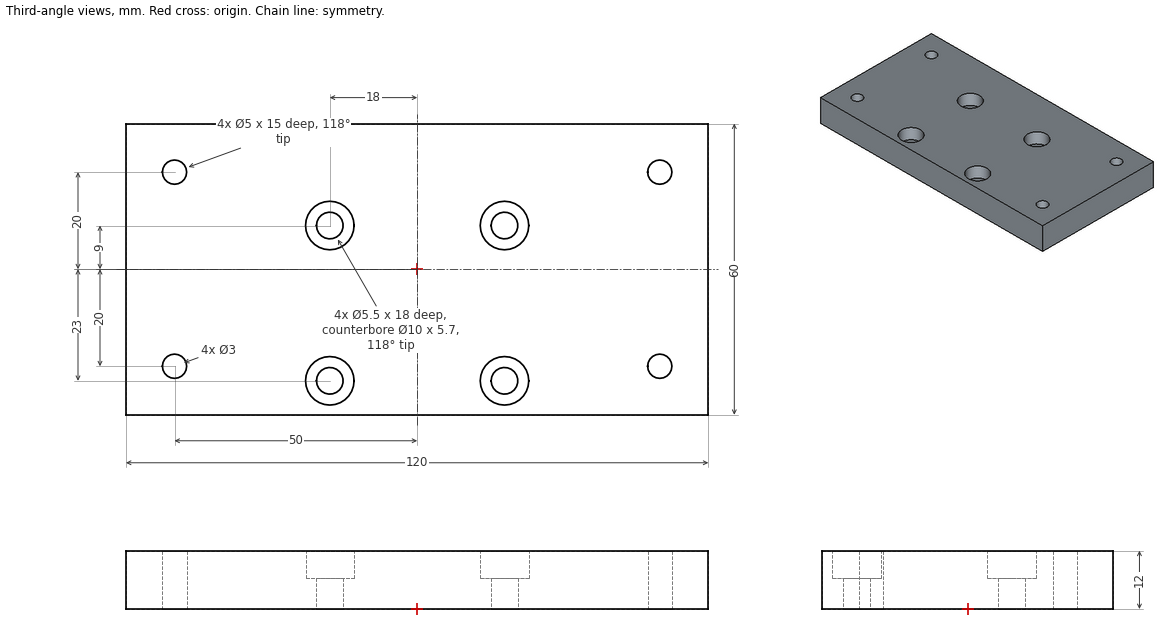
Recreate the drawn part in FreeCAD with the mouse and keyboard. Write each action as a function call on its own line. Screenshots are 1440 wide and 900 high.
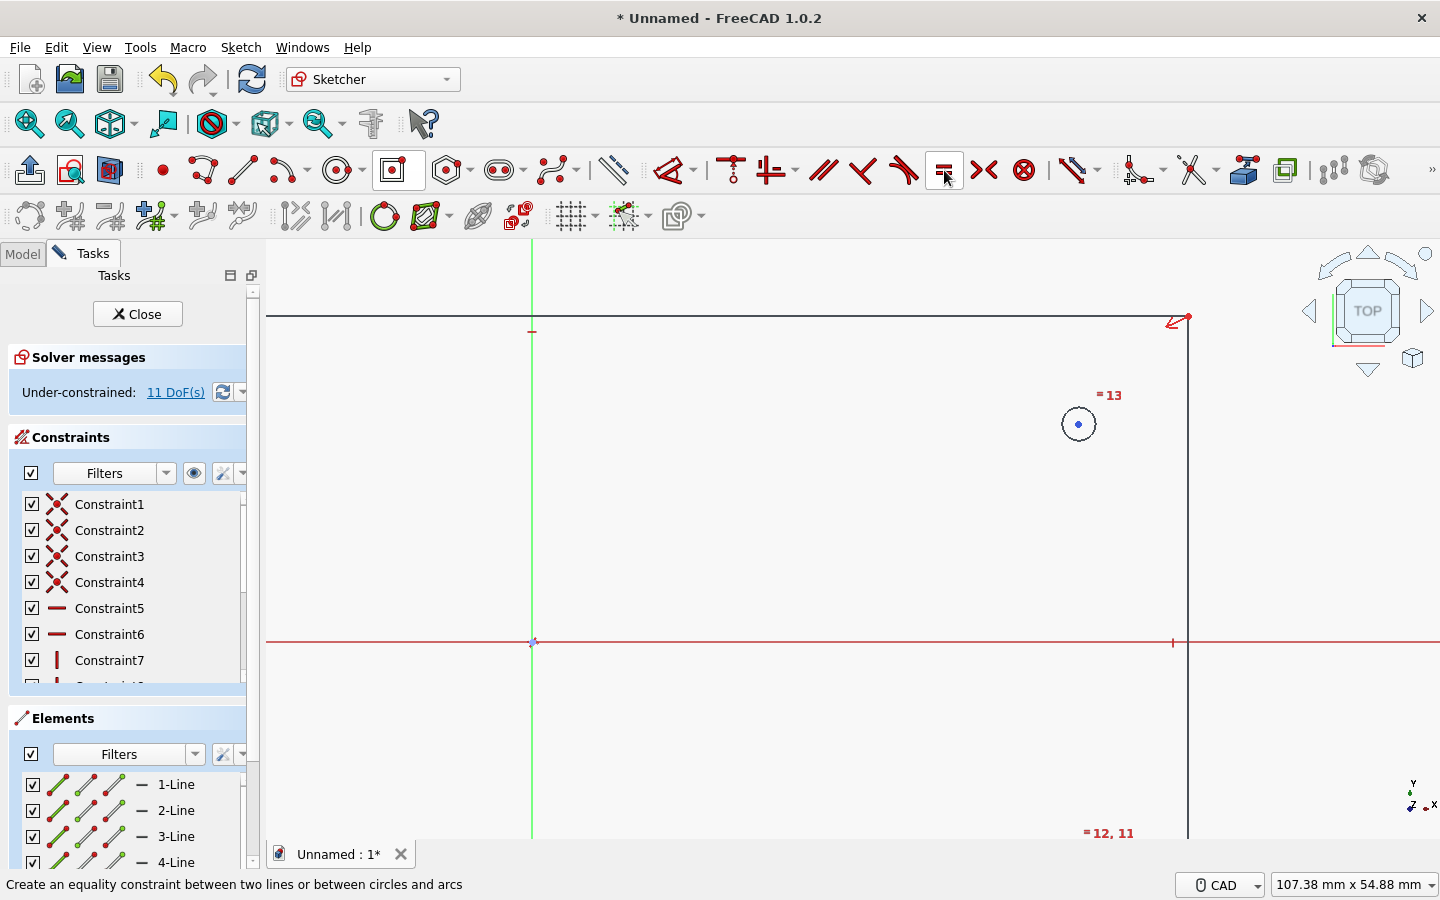
scroll(1091, 413, down, 3)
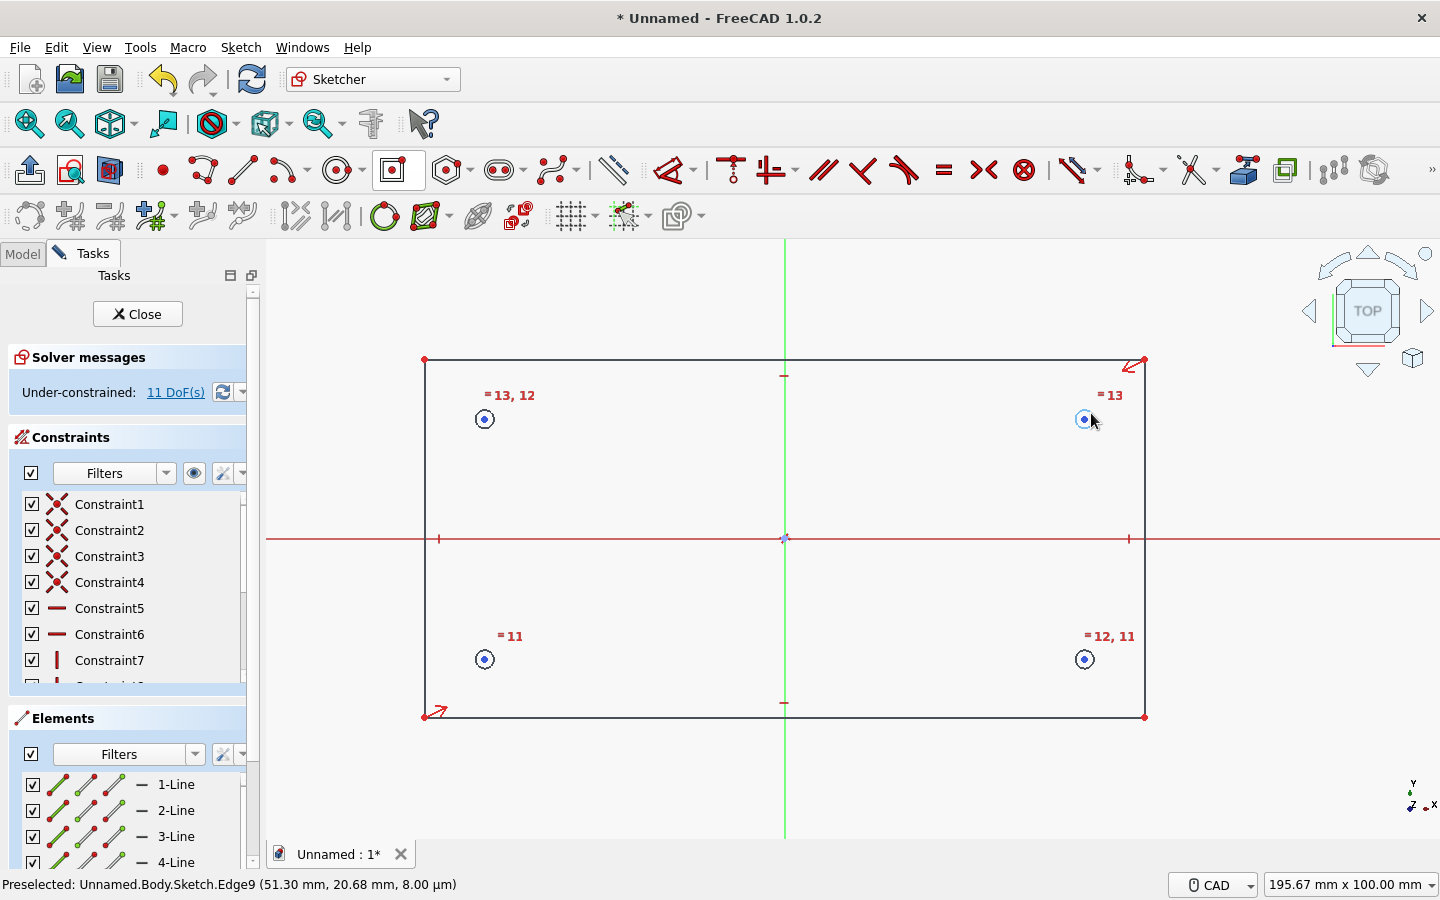
click(485, 659)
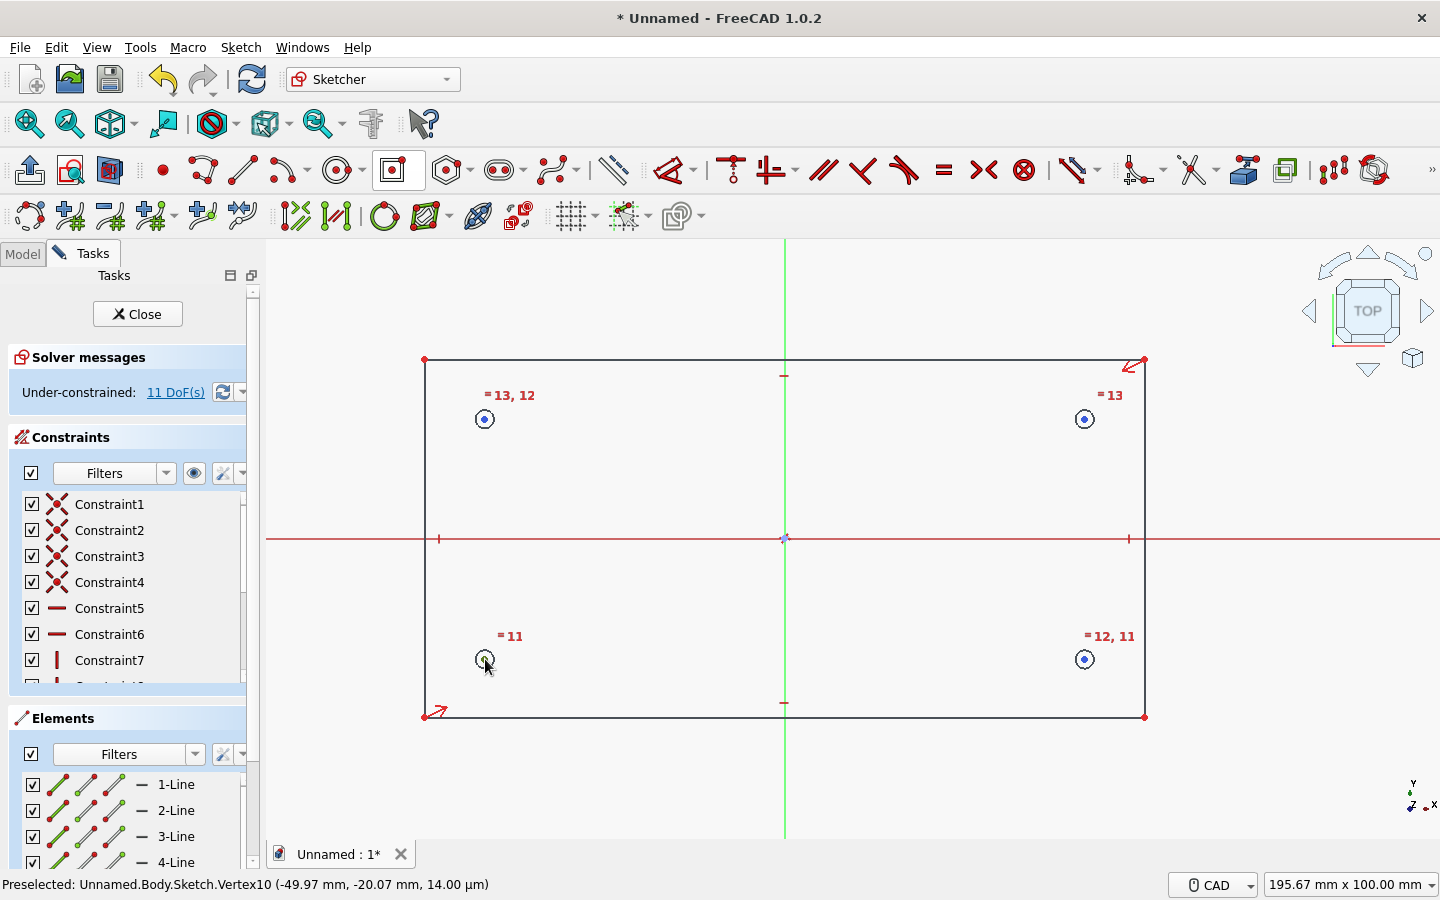
click(1085, 659)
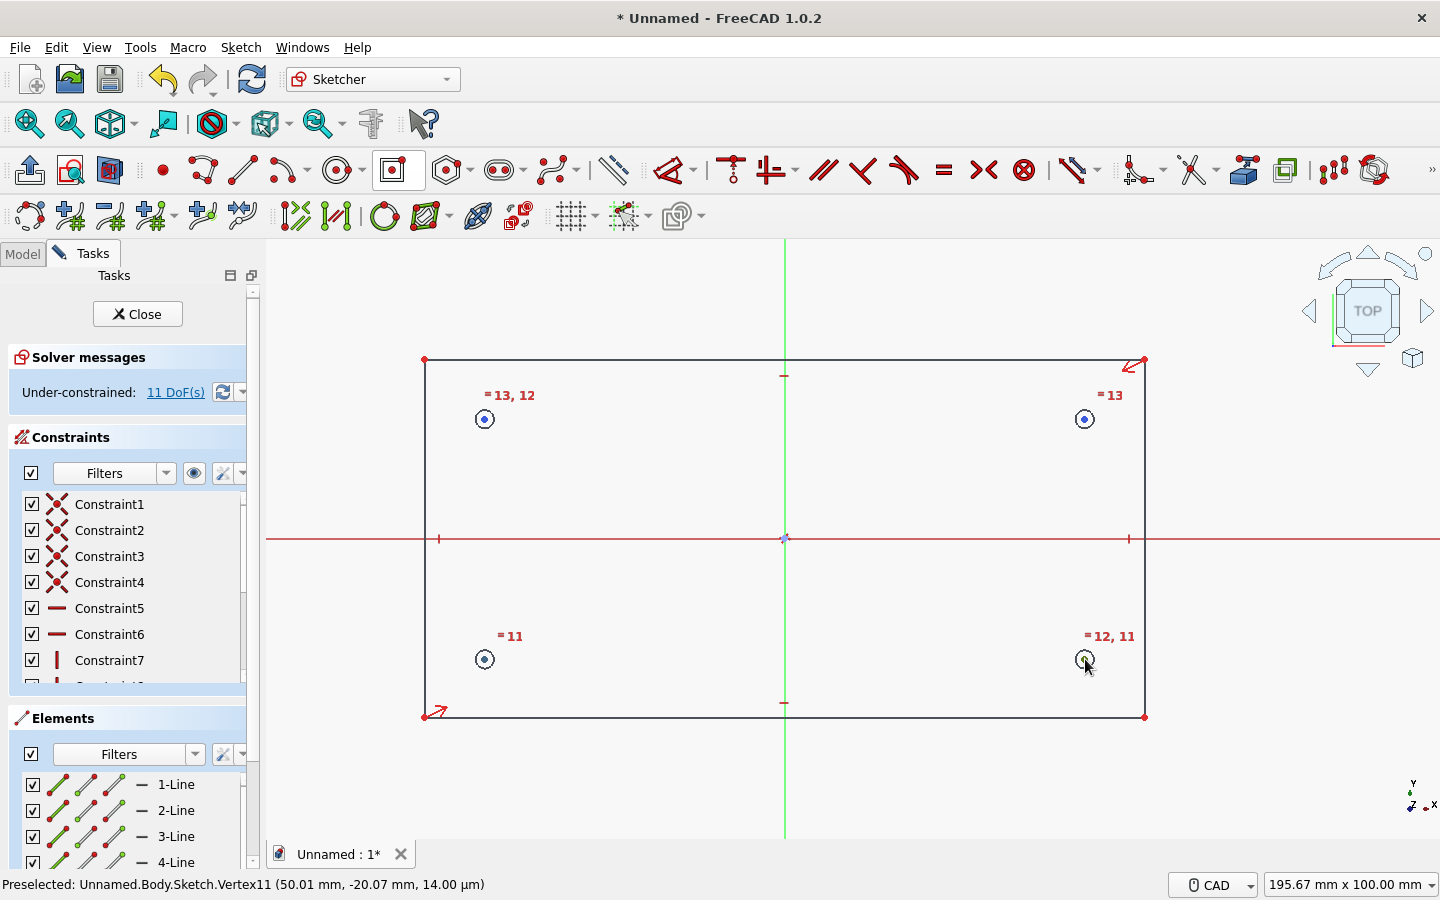
click(785, 772)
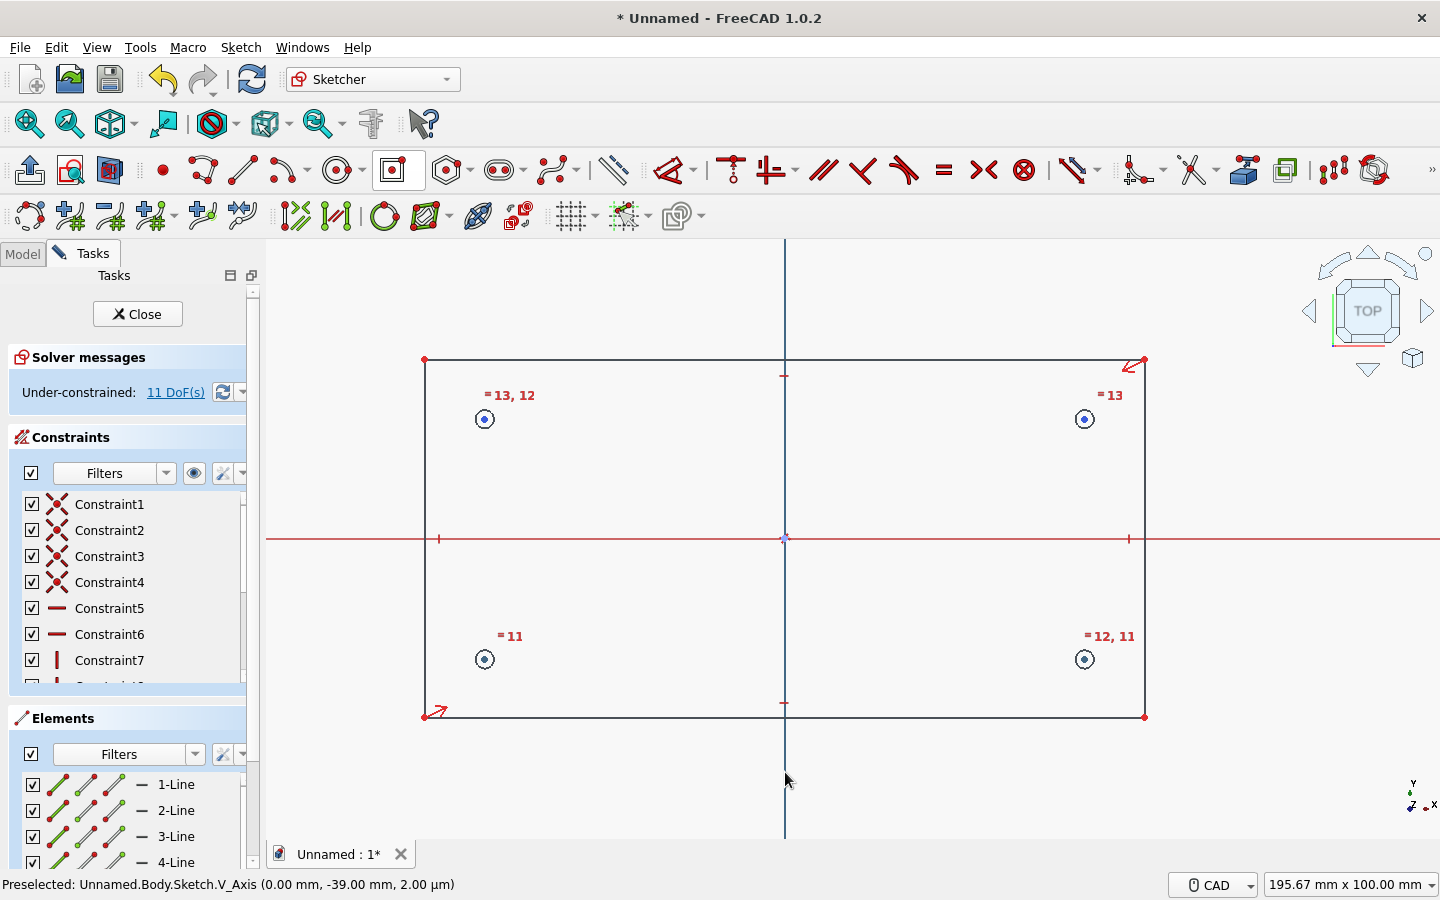
click(984, 170)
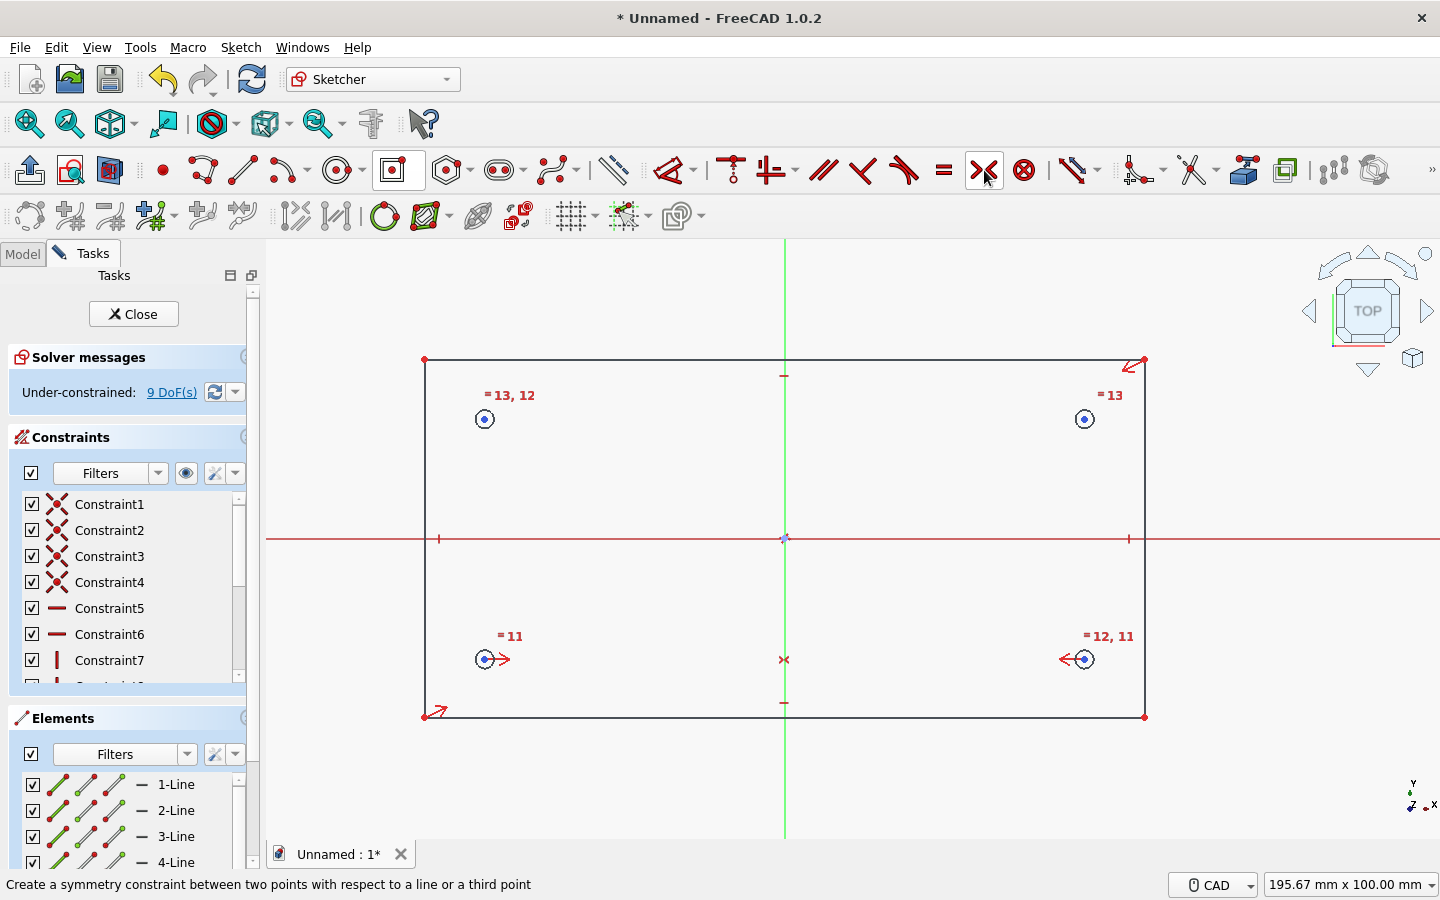
click(485, 659)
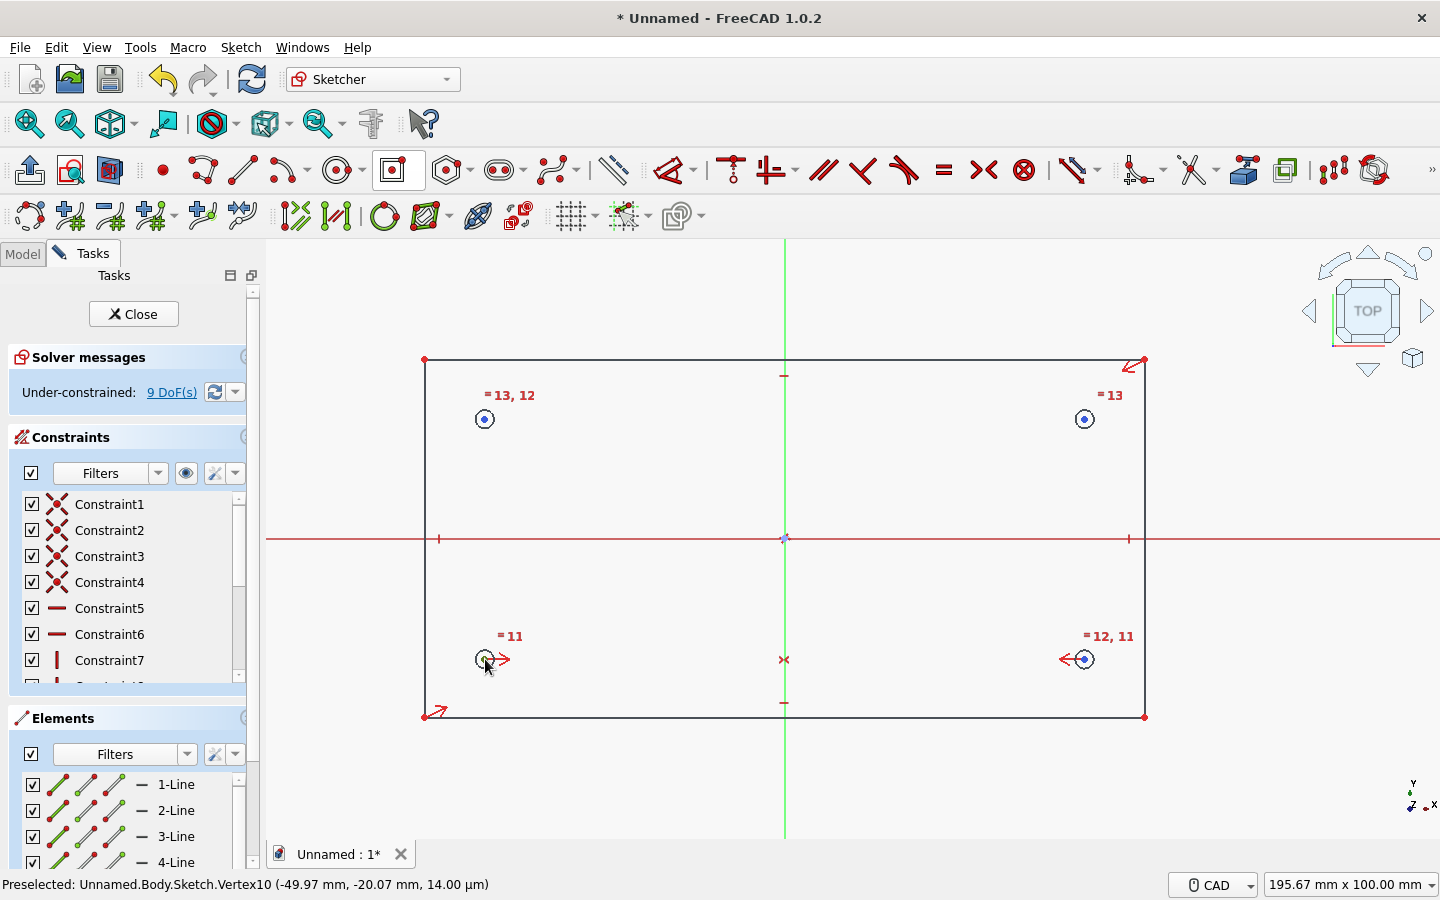
click(485, 419)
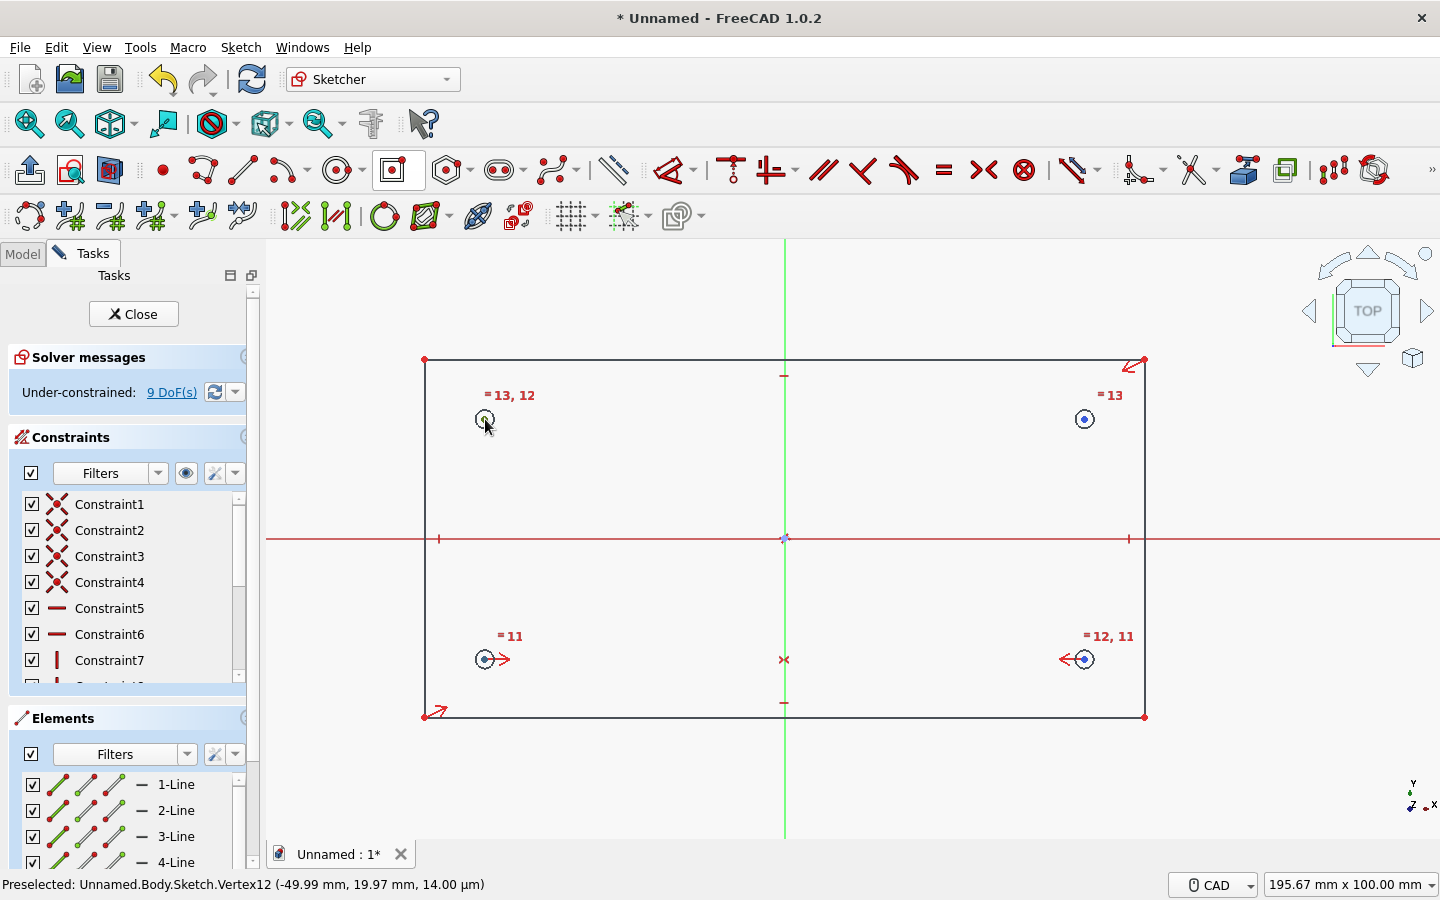
click(364, 539)